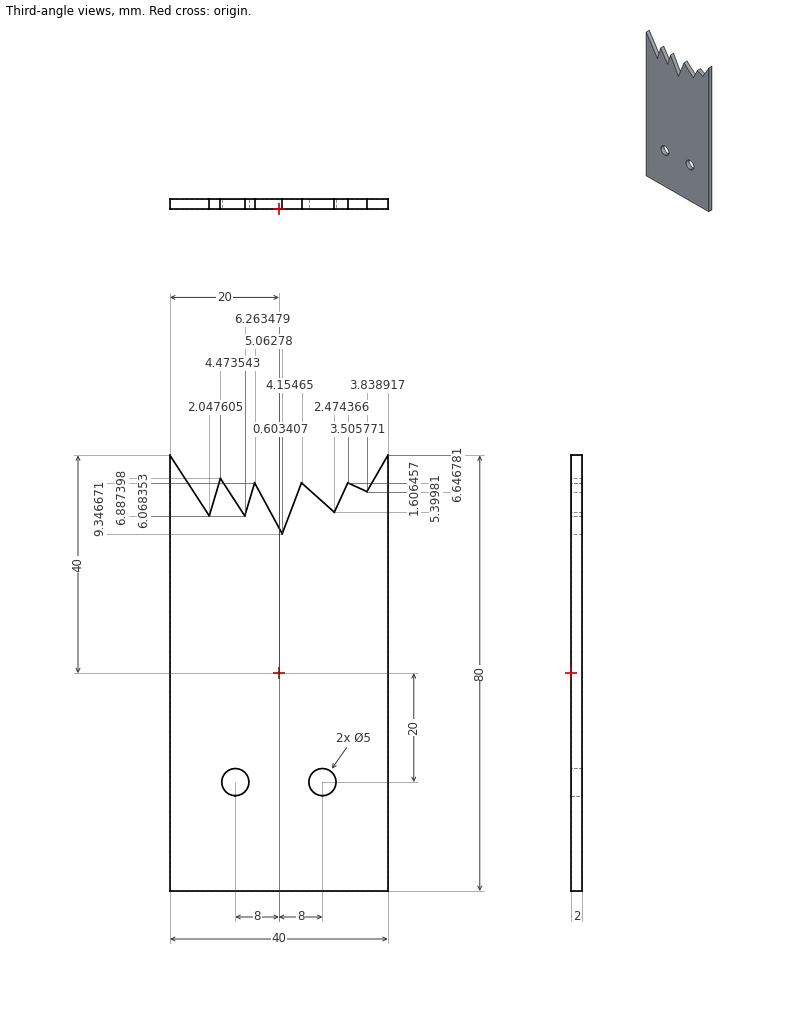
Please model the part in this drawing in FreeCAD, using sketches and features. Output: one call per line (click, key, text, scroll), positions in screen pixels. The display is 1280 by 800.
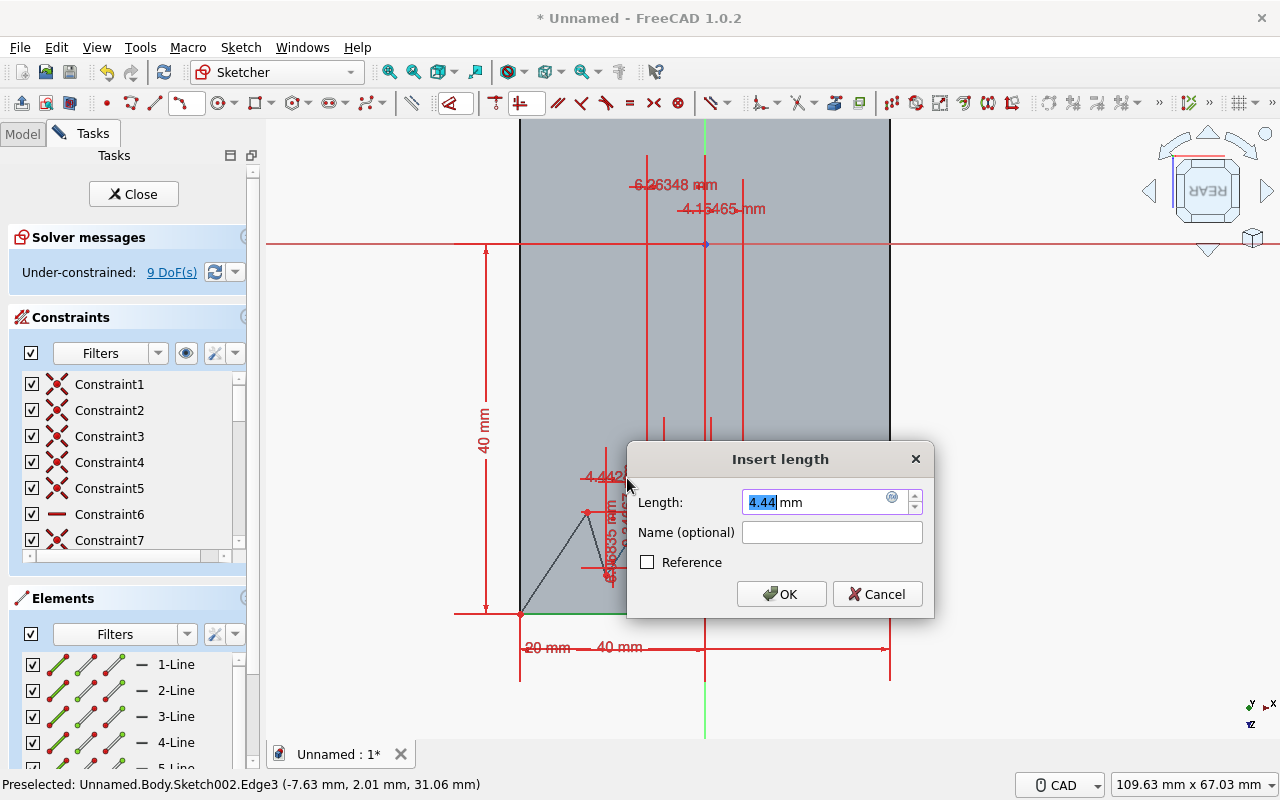
text(4.473543)
key(Return)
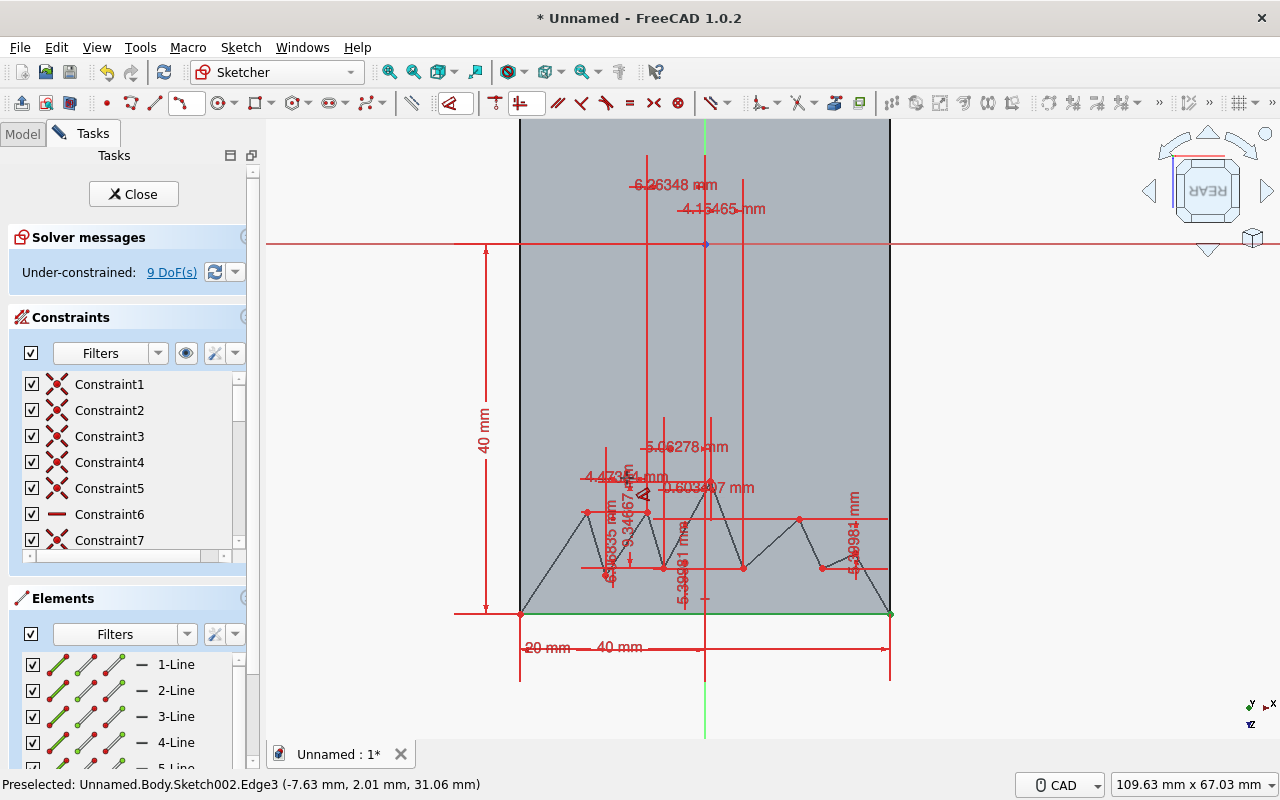
click(635, 531)
click(572, 566)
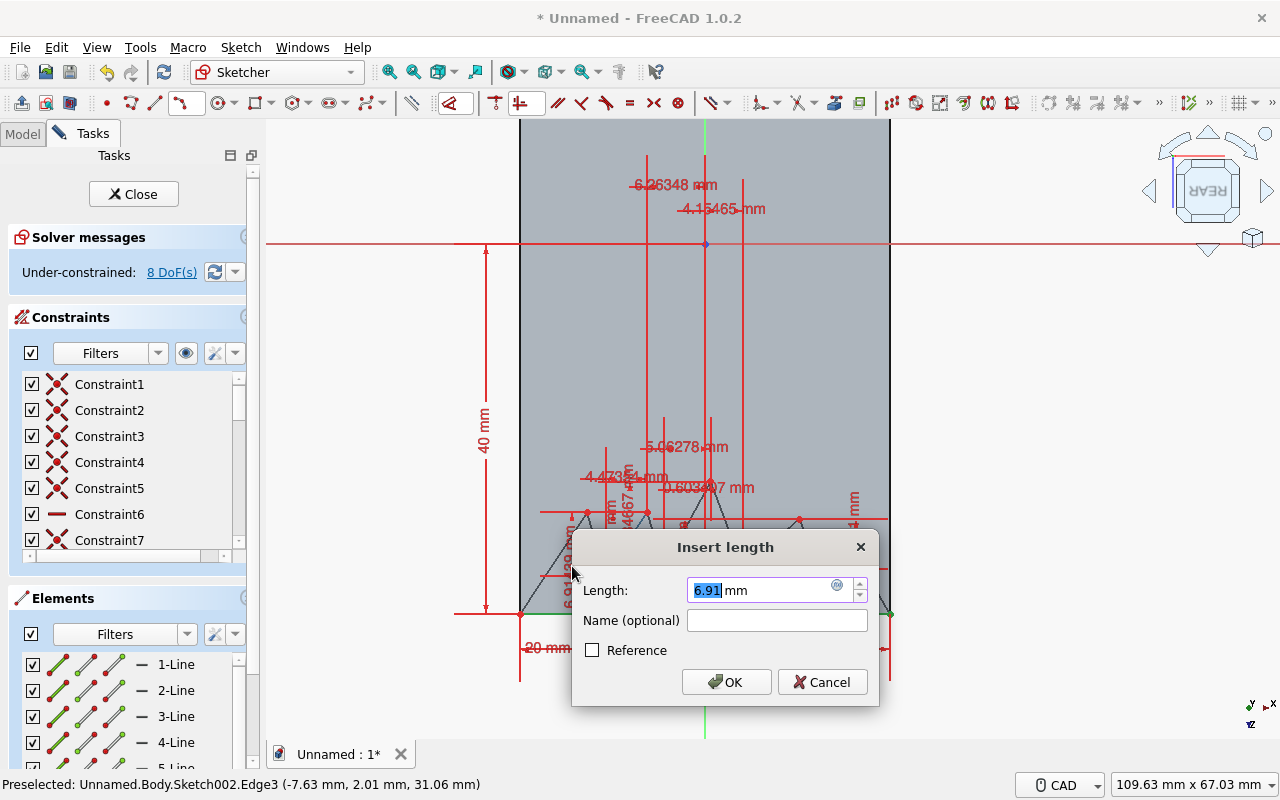
text(6.887398)
key(Return)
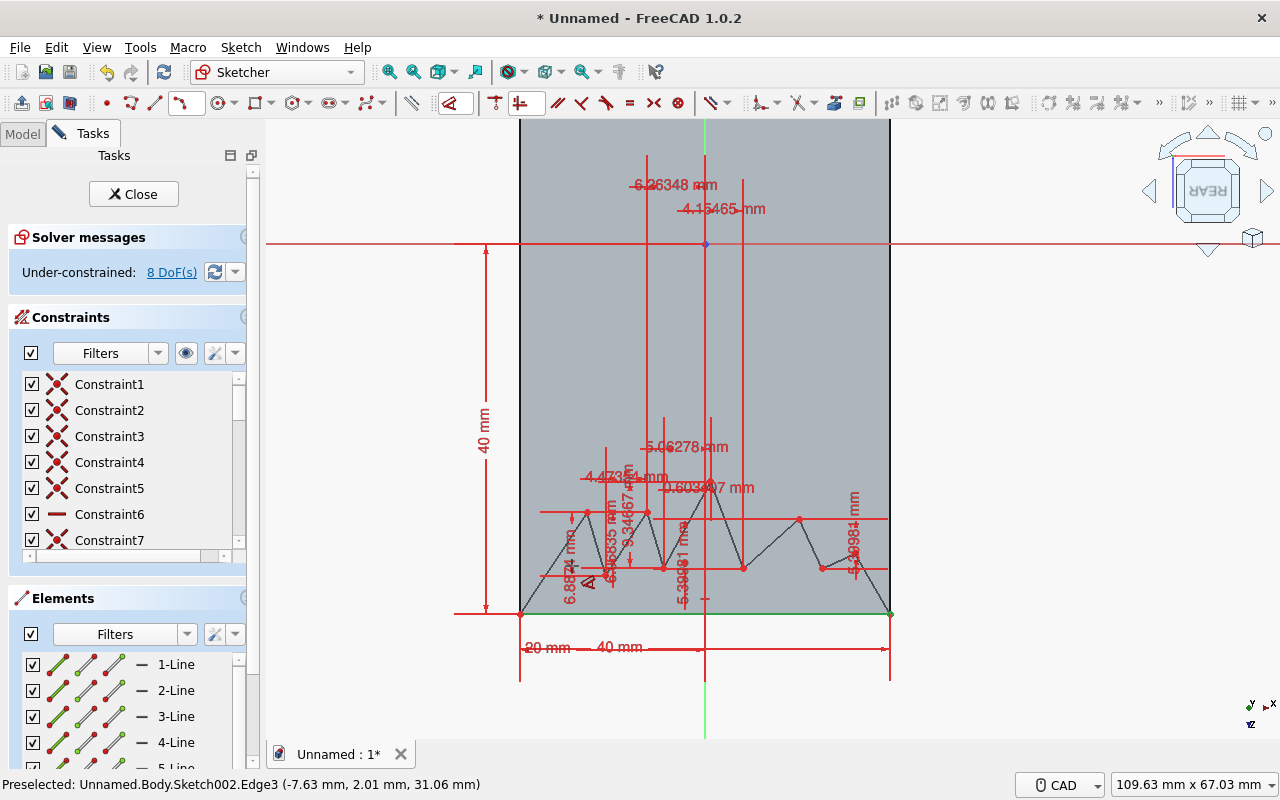
scroll(600, 557, up, 4)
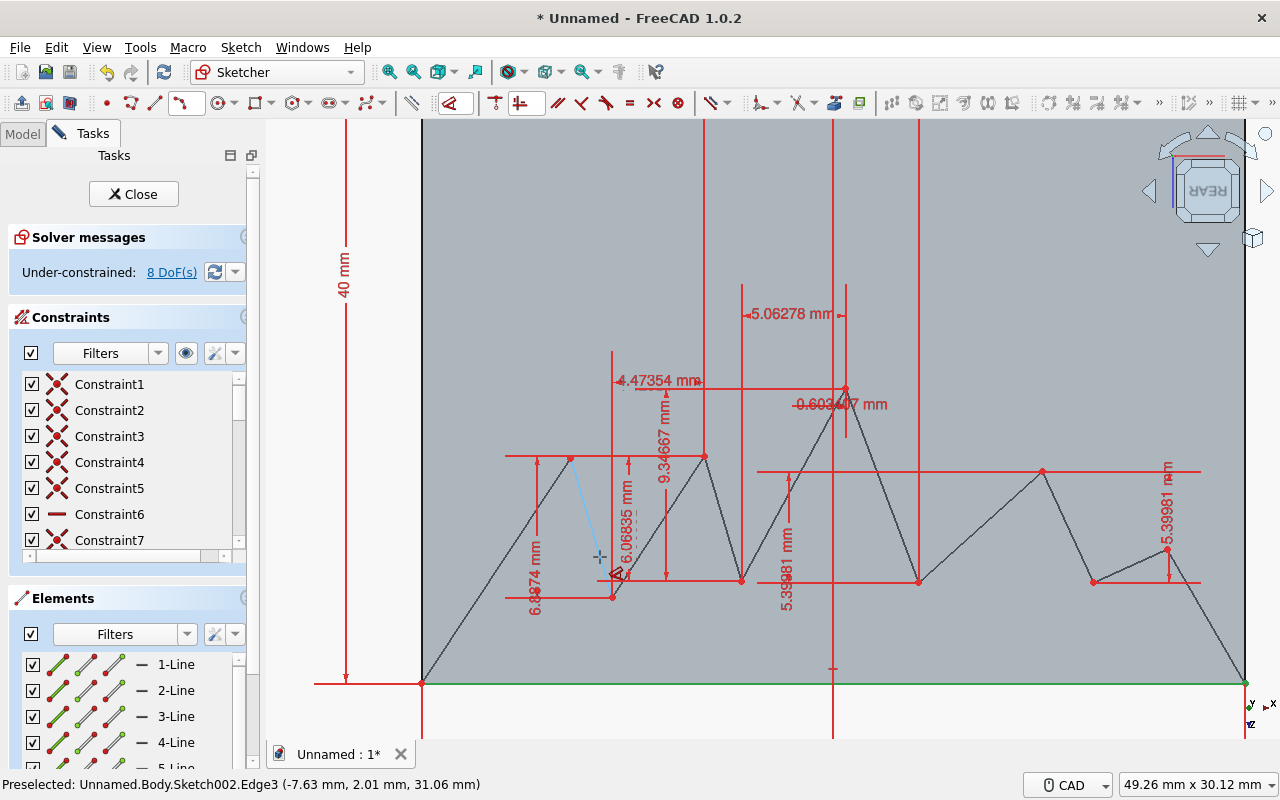
click(600, 556)
click(591, 632)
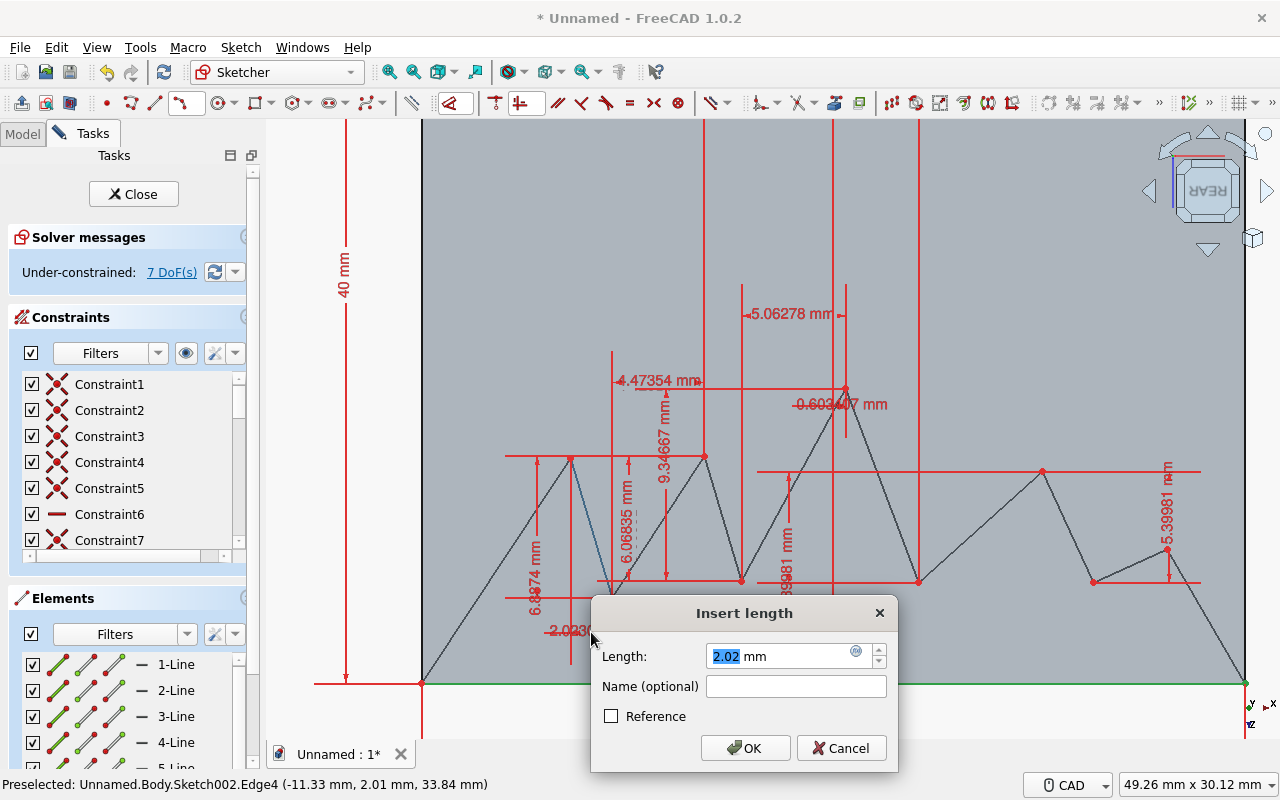
text(2.047605)
key(Return)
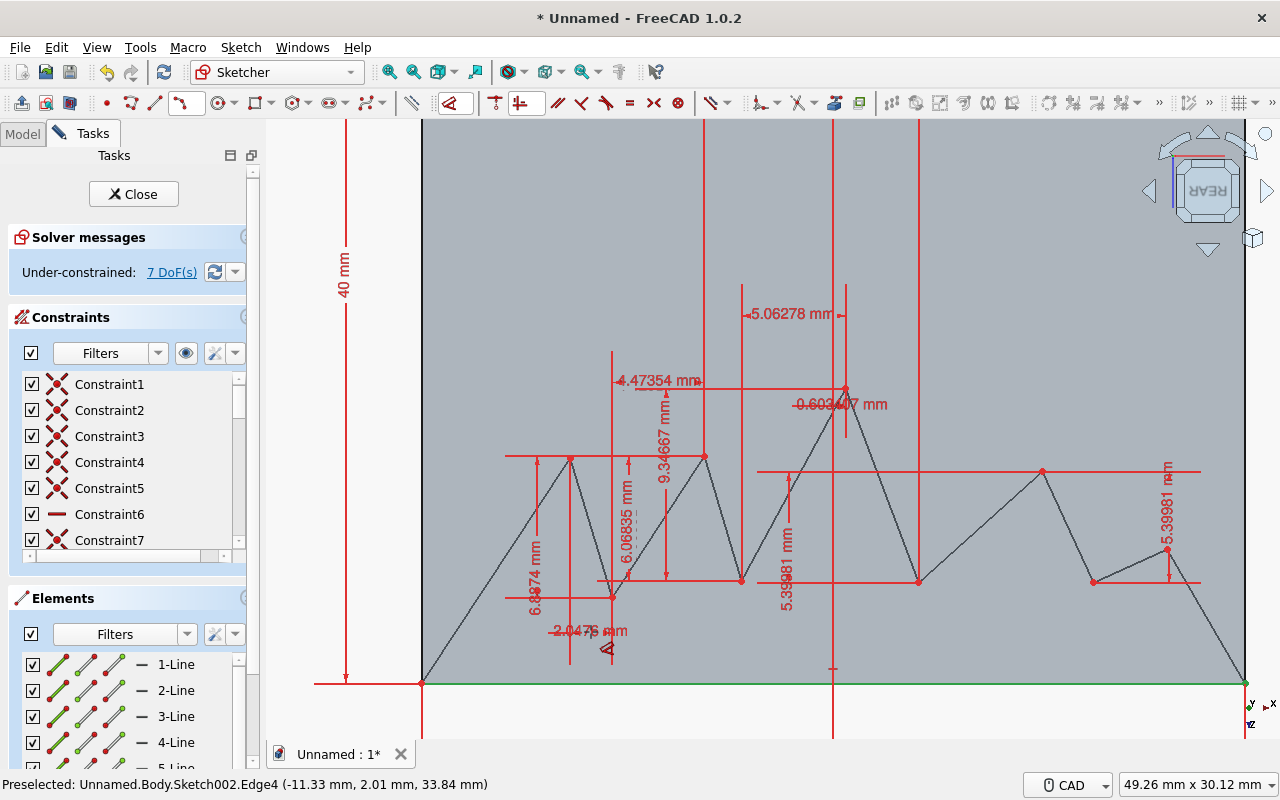
click(600, 556)
click(536, 479)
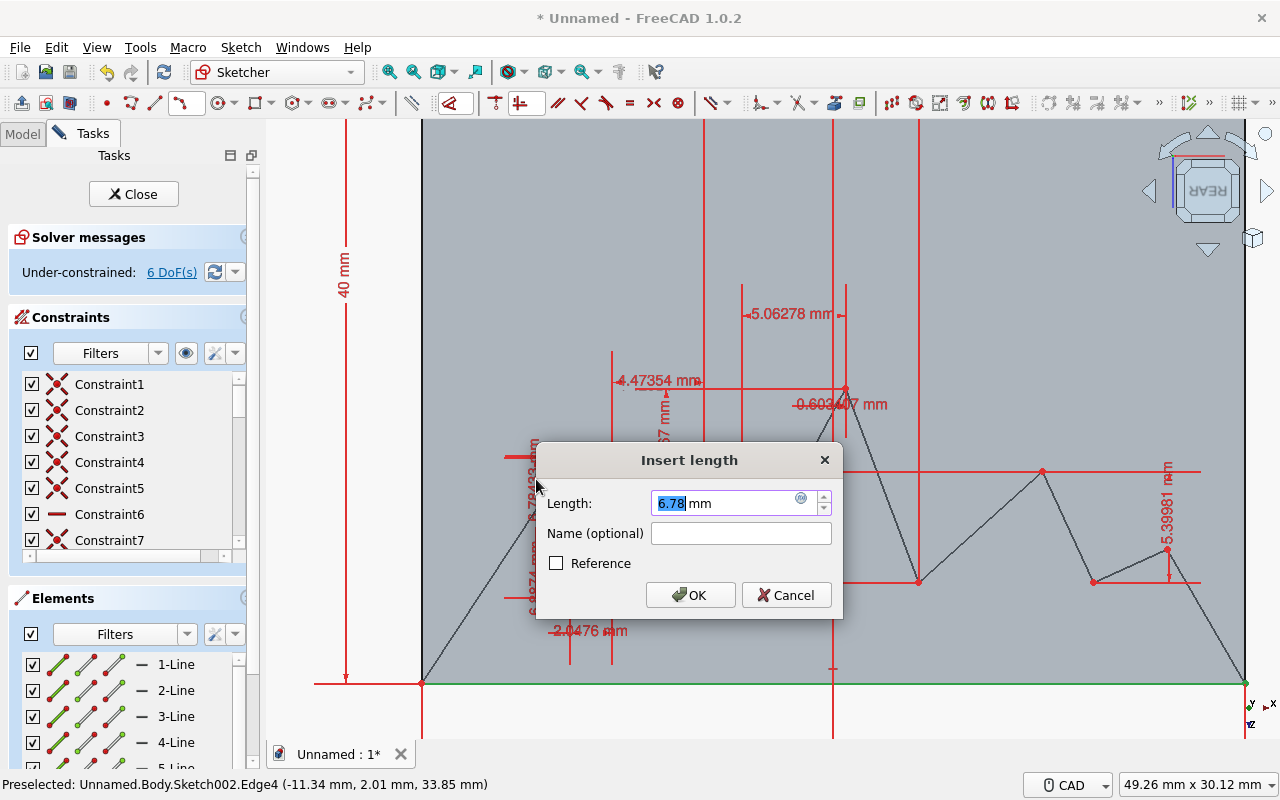
text(6.887398)
key(Return)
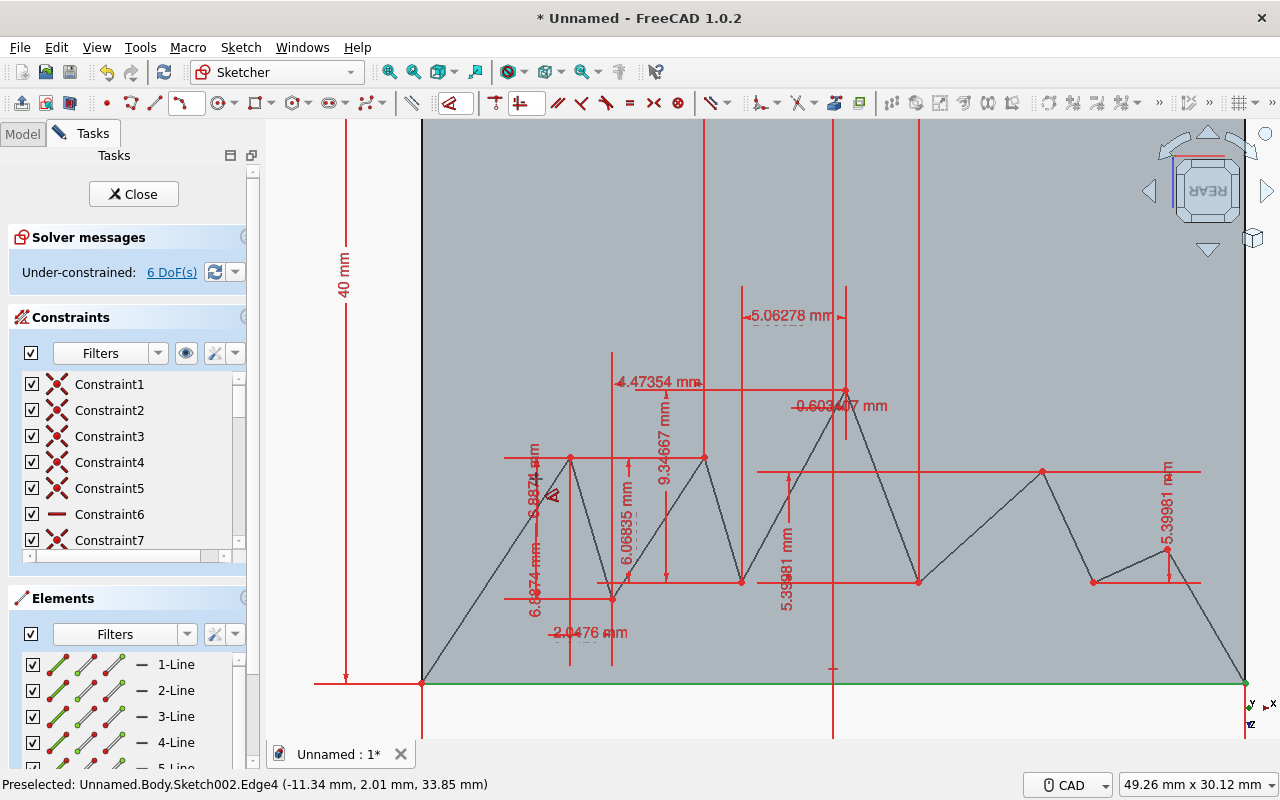
scroll(599, 557, down, 4)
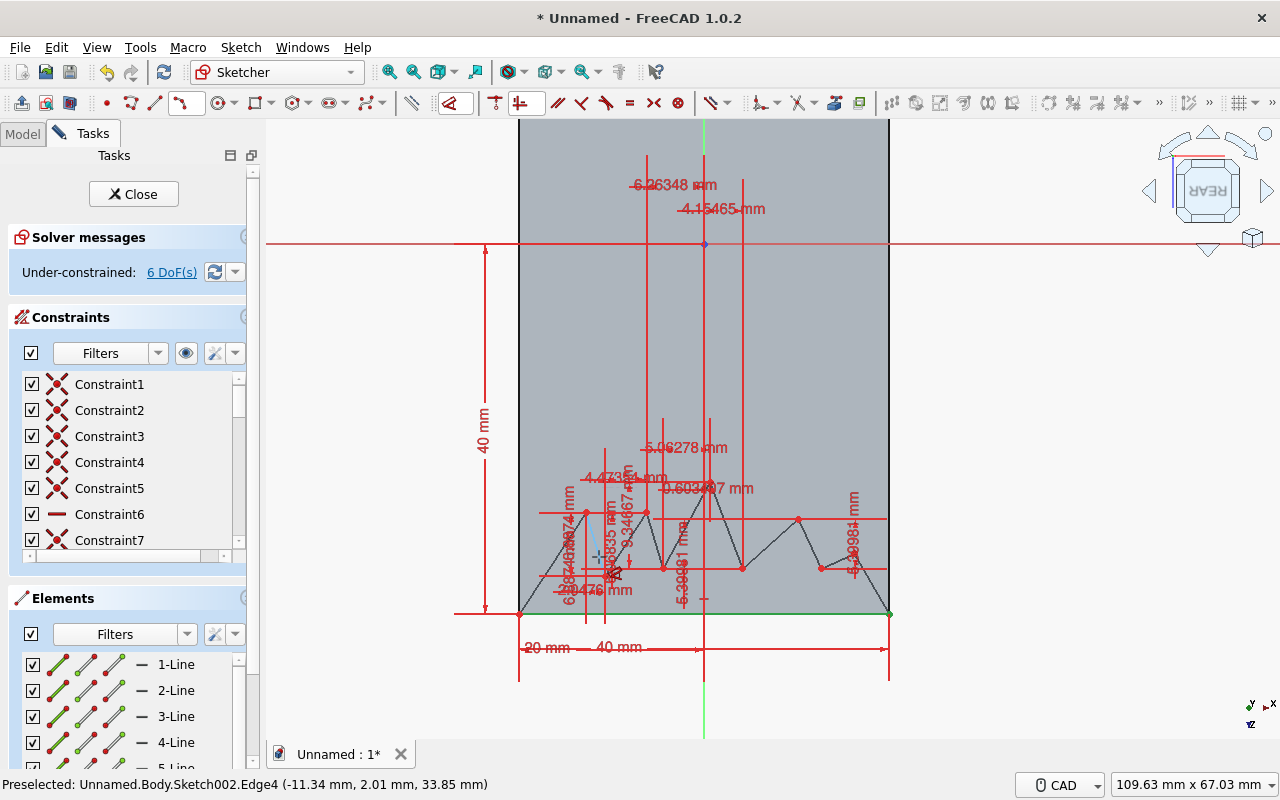
click(879, 596)
click(872, 648)